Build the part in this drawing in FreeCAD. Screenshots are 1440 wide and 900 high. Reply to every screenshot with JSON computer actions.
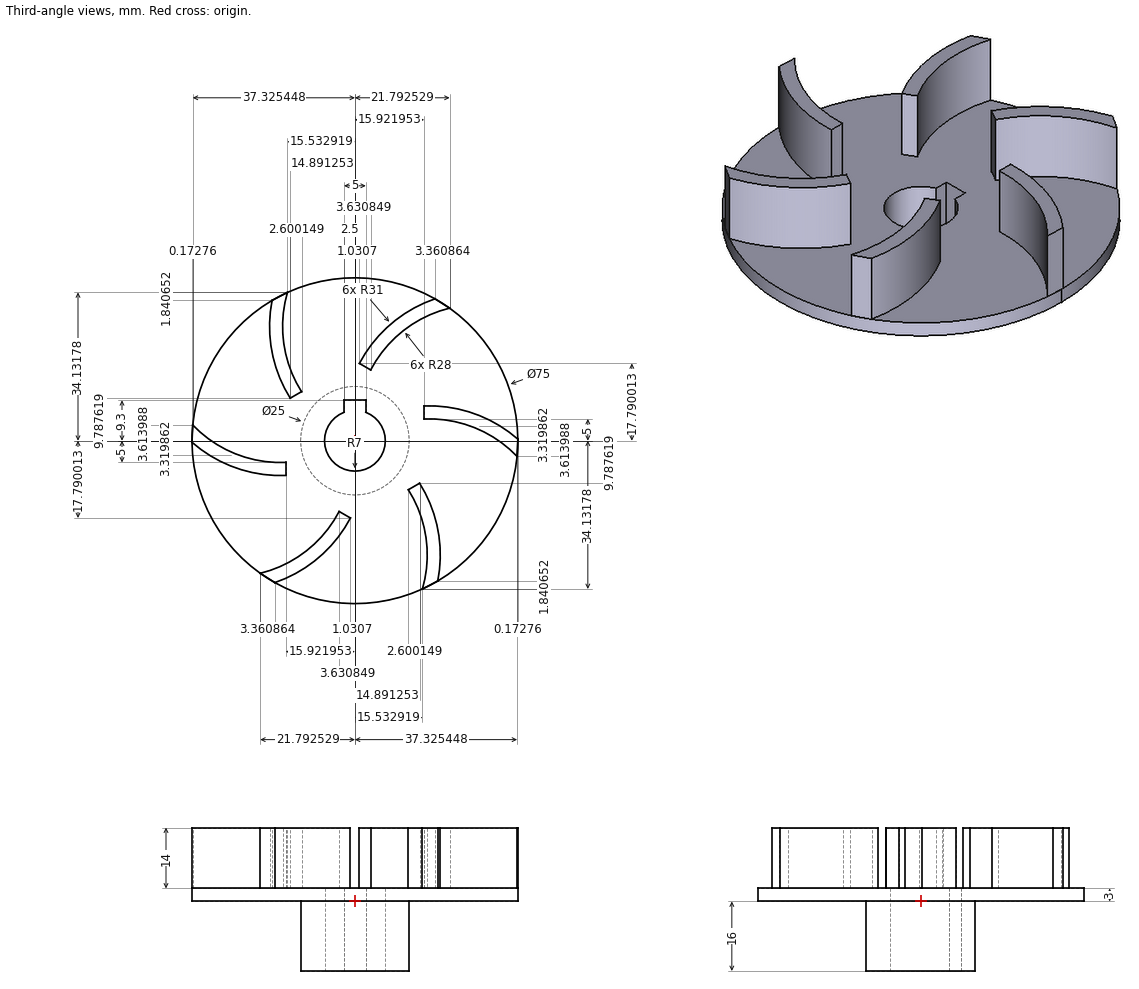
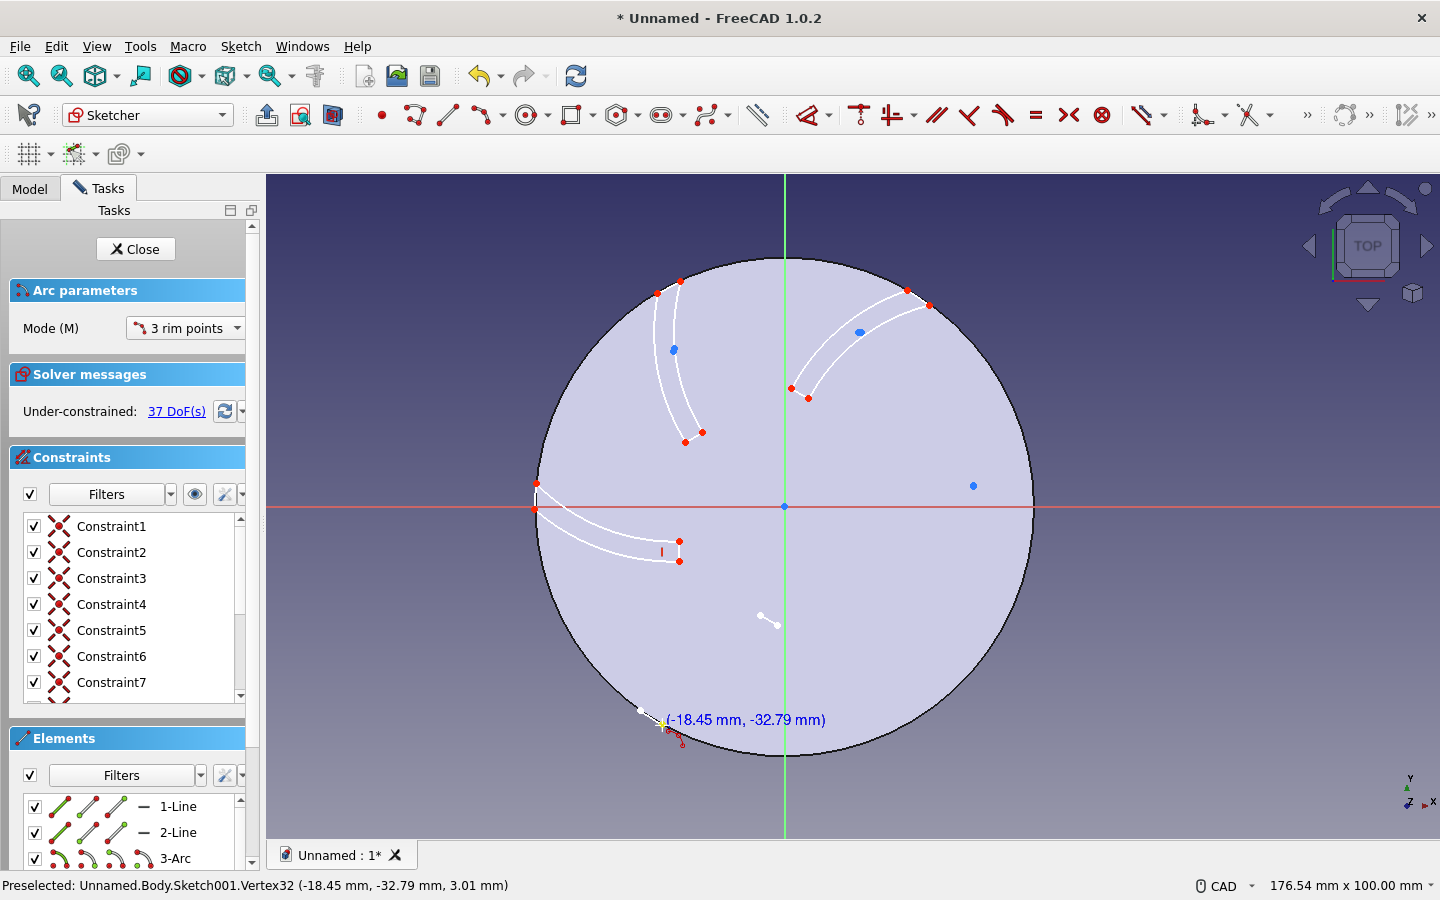
{"action": "scroll", "coordinate": [778, 625], "scroll_direction": "up", "scroll_amount": 5}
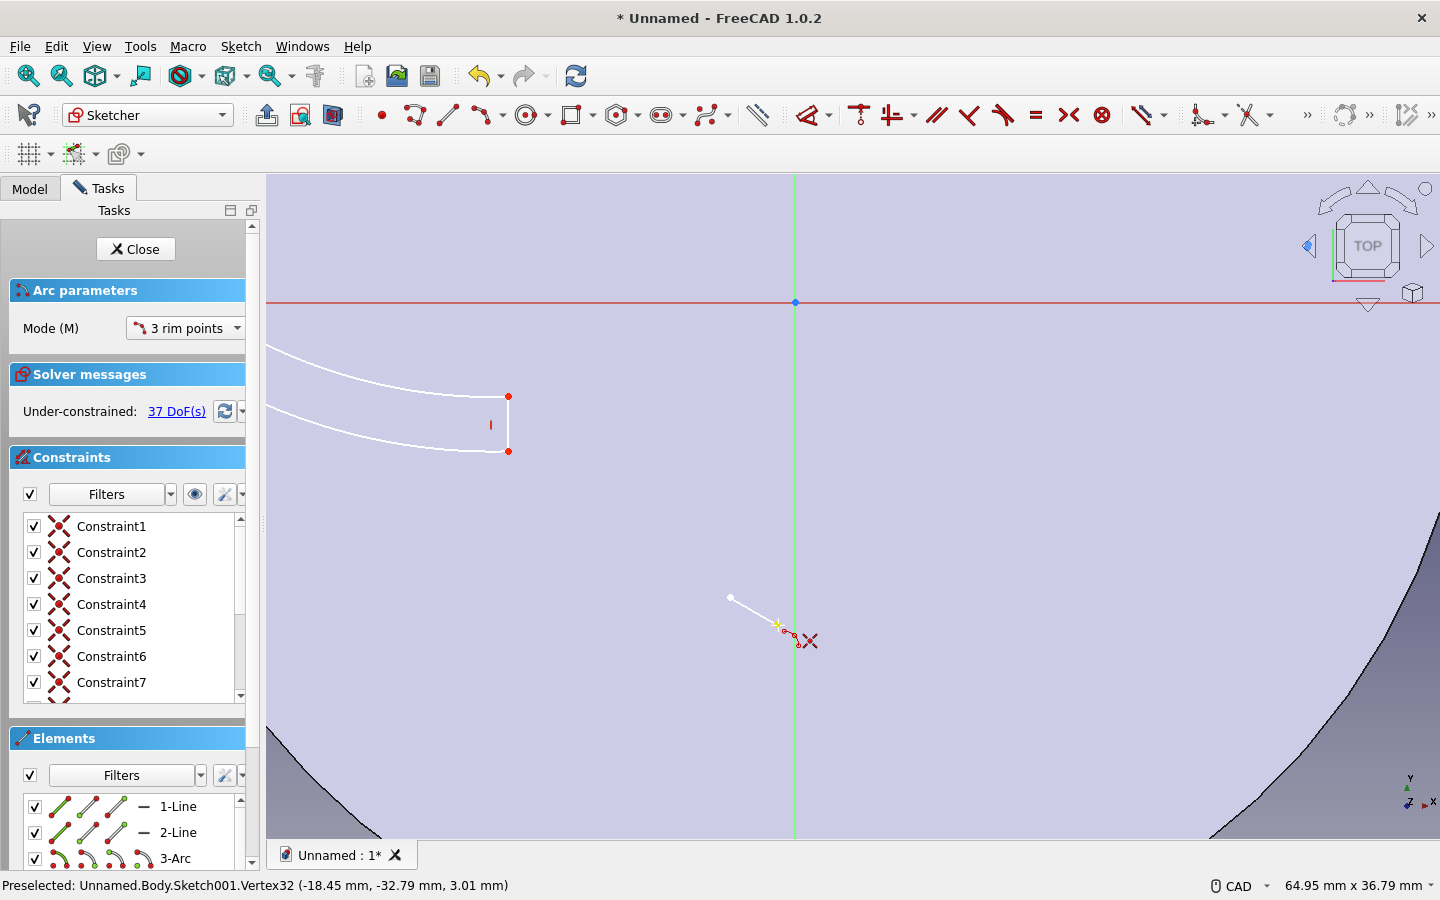
{"action": "left_click", "coordinate": [777, 625]}
{"action": "left_click", "coordinate": [645, 789]}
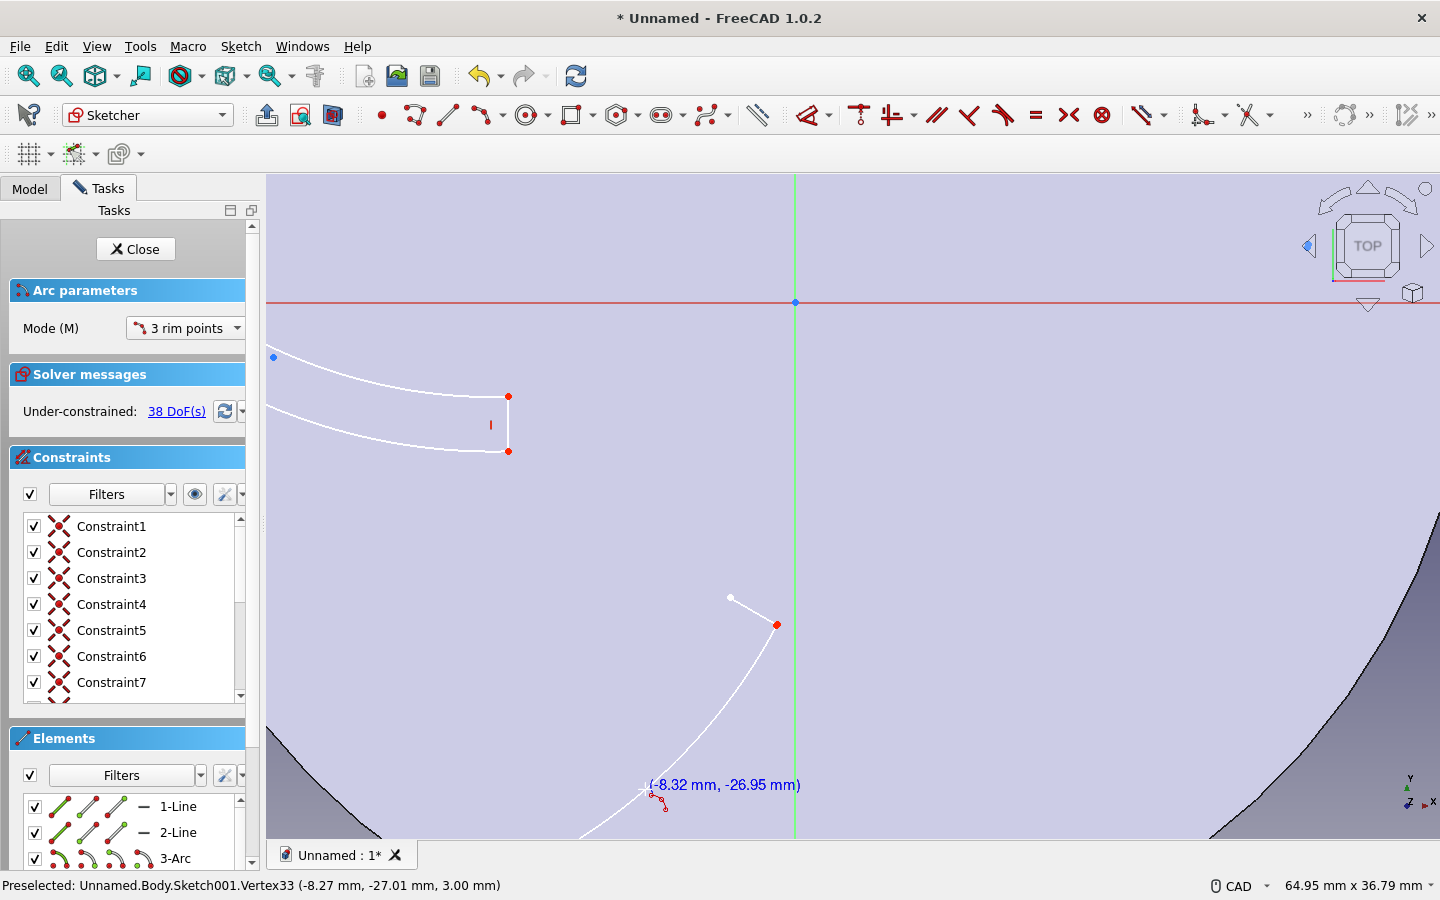
{"action": "left_click", "coordinate": [730, 598]}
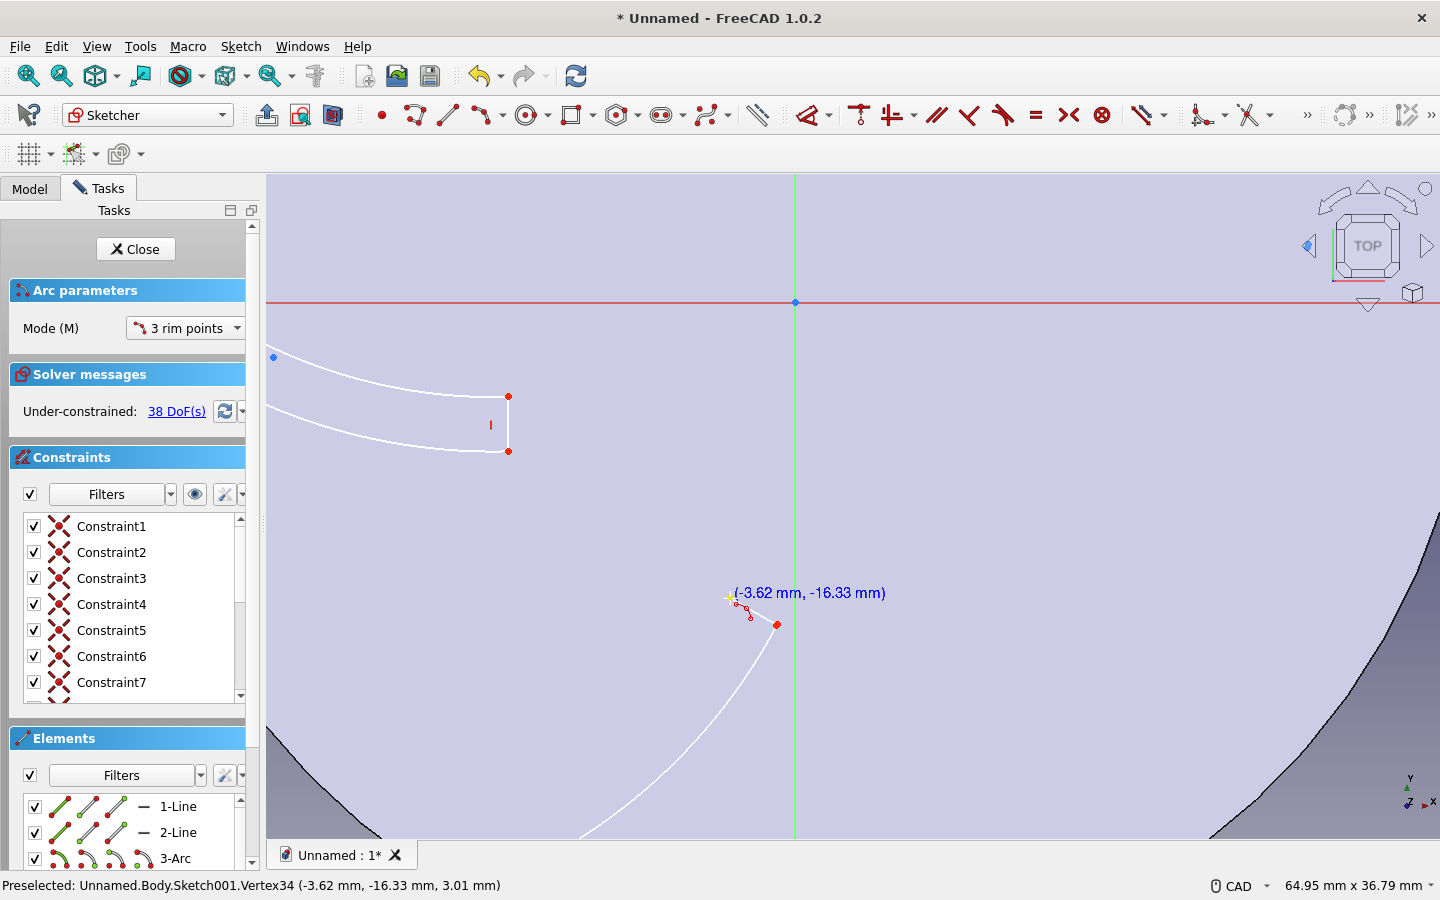
{"action": "scroll", "coordinate": [778, 625], "scroll_direction": "down", "scroll_amount": 5}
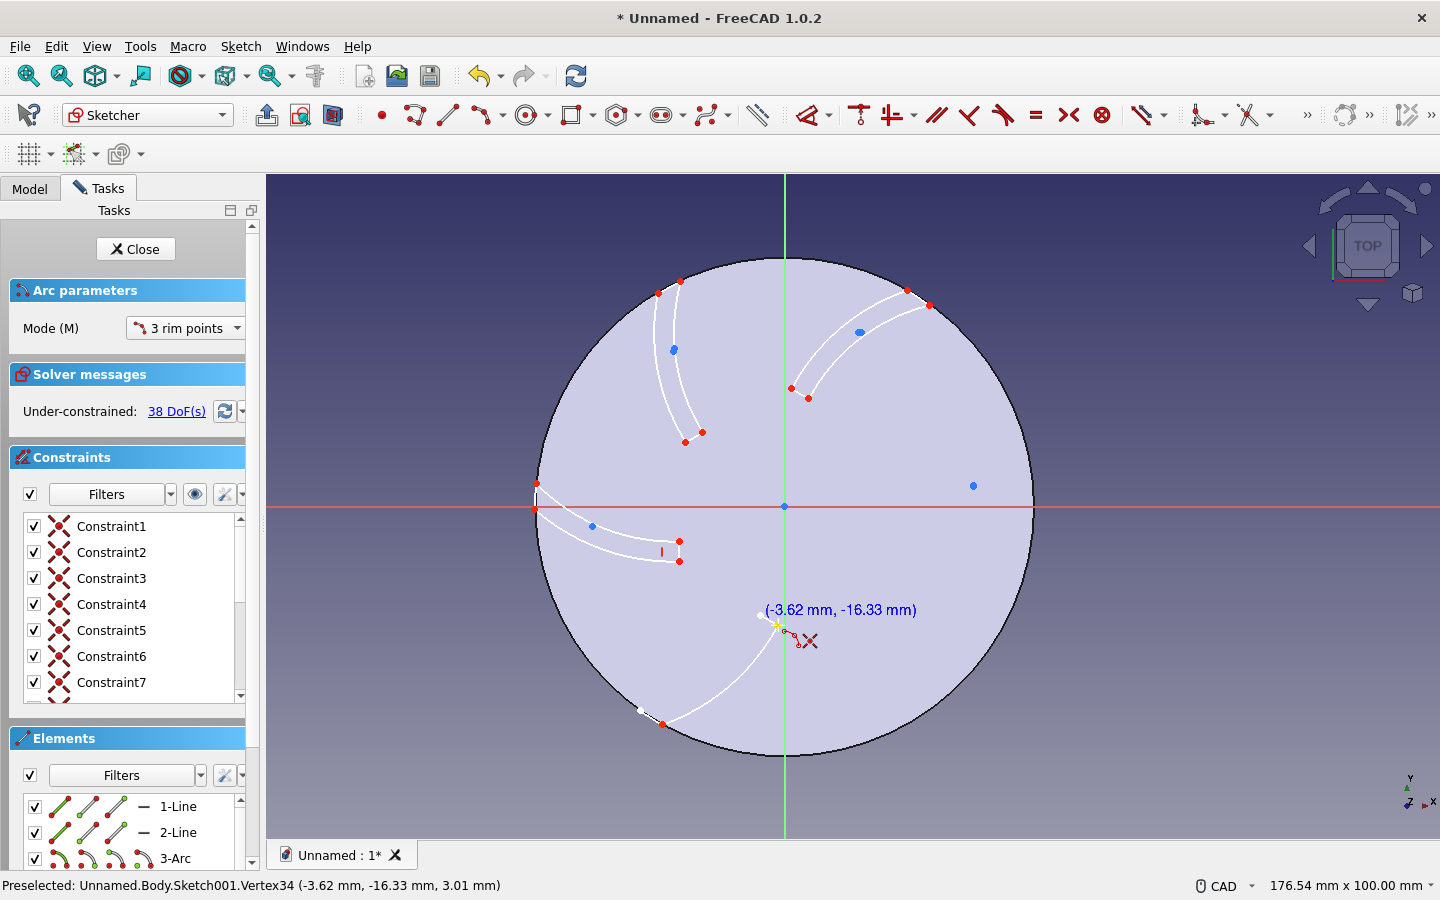
{"action": "left_click", "coordinate": [640, 711]}
{"action": "left_click", "coordinate": [710, 676]}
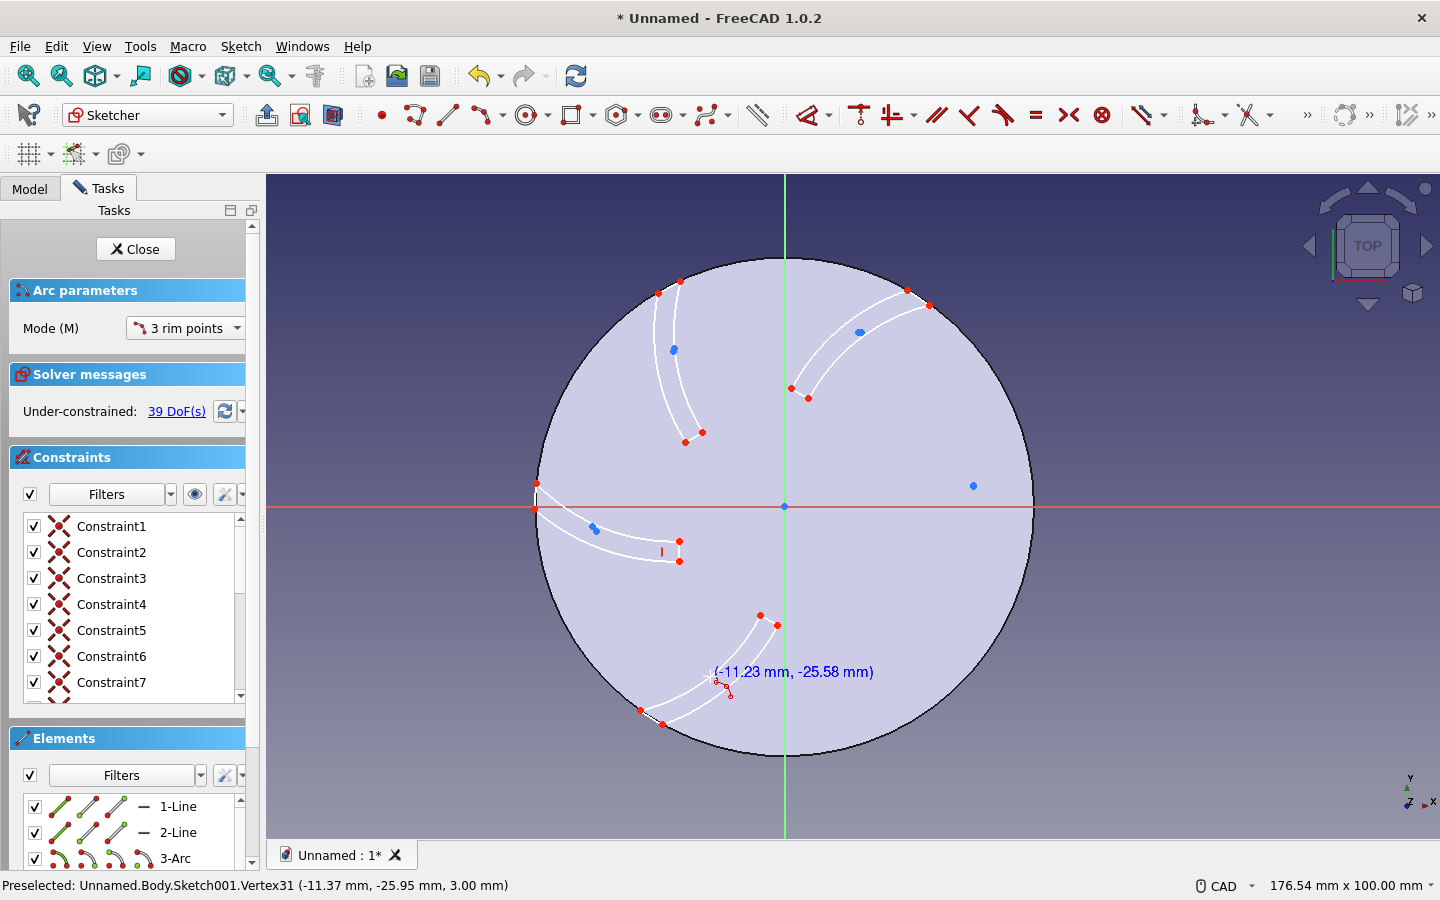
{"action": "key", "text": "g l"}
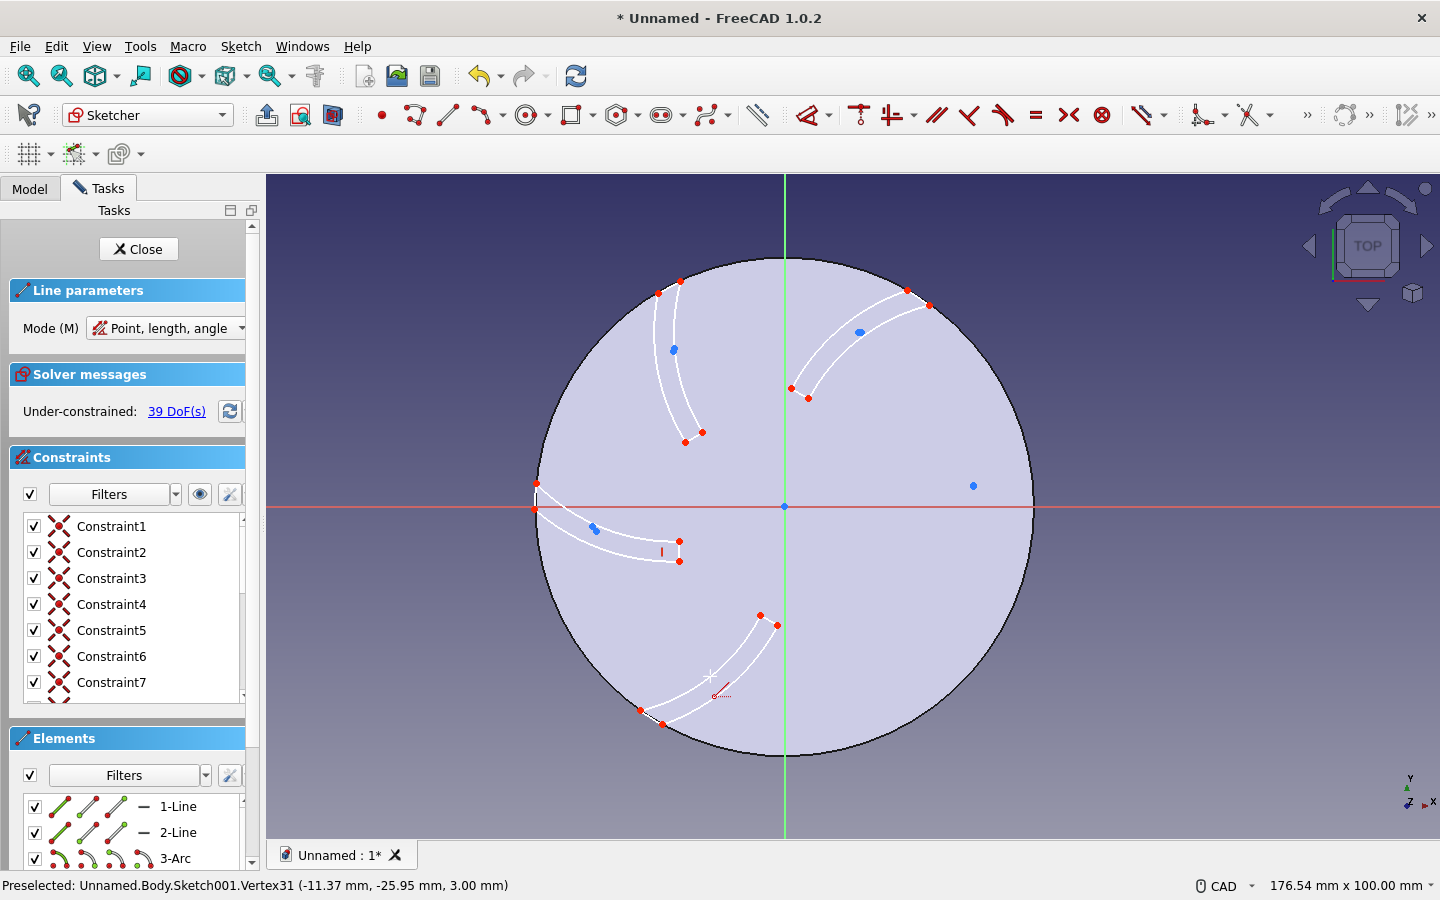
{"action": "left_click", "coordinate": [888, 734]}
{"action": "left_click", "coordinate": [911, 722]}